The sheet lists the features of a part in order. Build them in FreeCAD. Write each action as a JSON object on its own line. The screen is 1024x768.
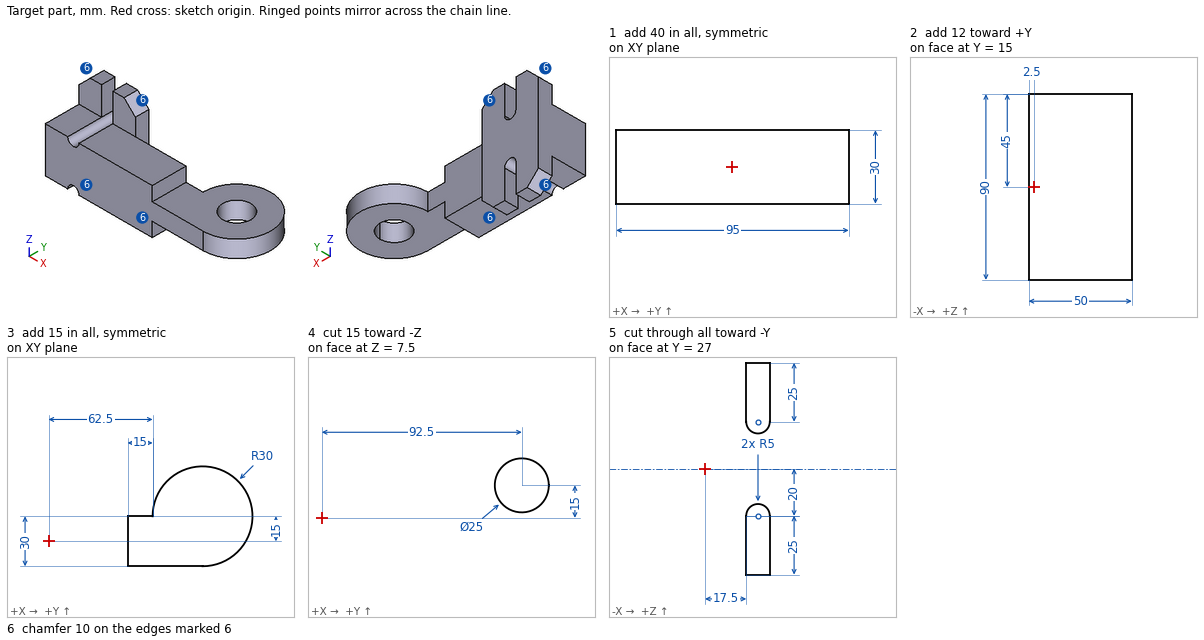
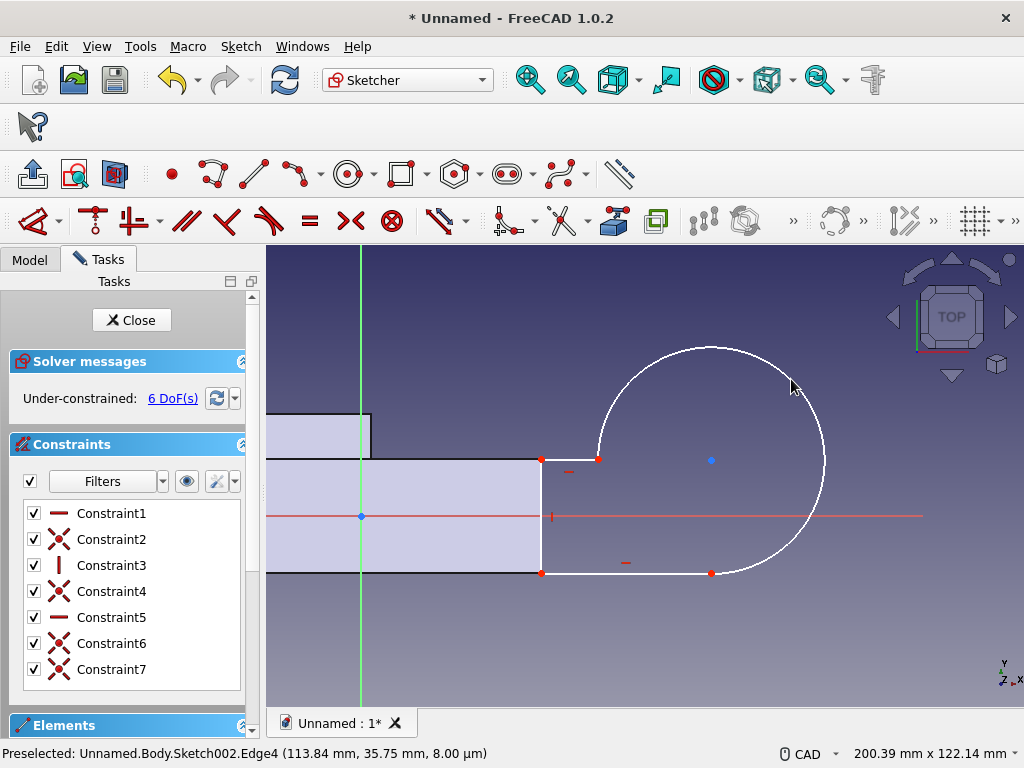
{"action": "left_click", "coordinate": [592, 574]}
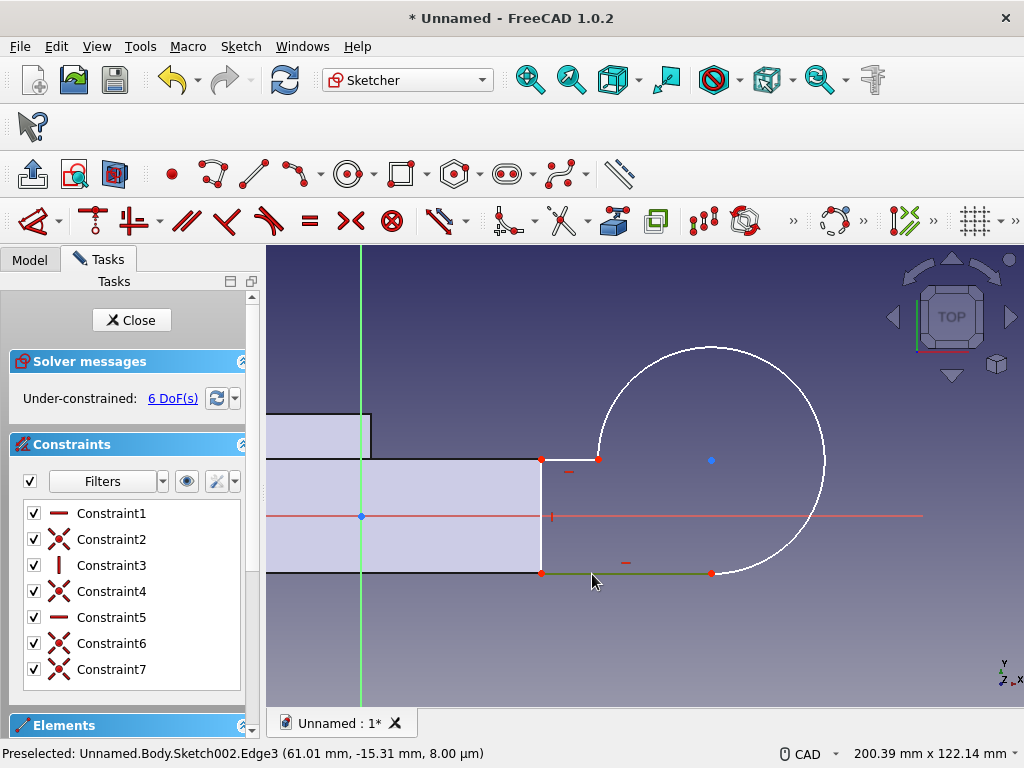
{"action": "left_click", "coordinate": [823, 479]}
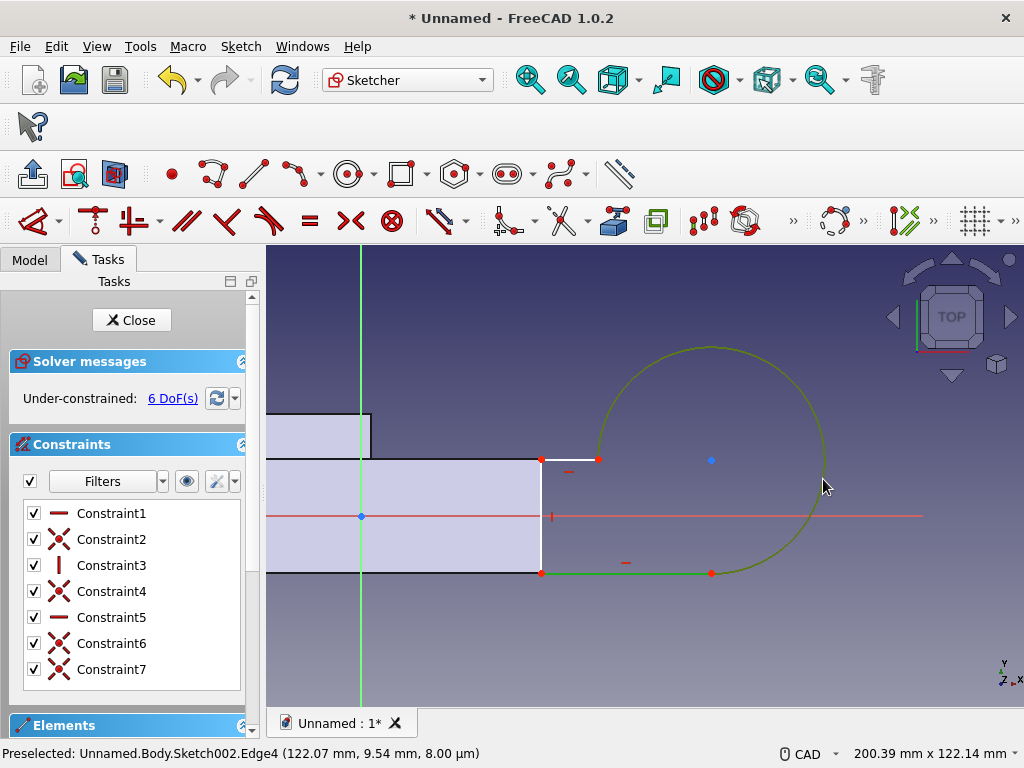
{"action": "left_click", "coordinate": [269, 222]}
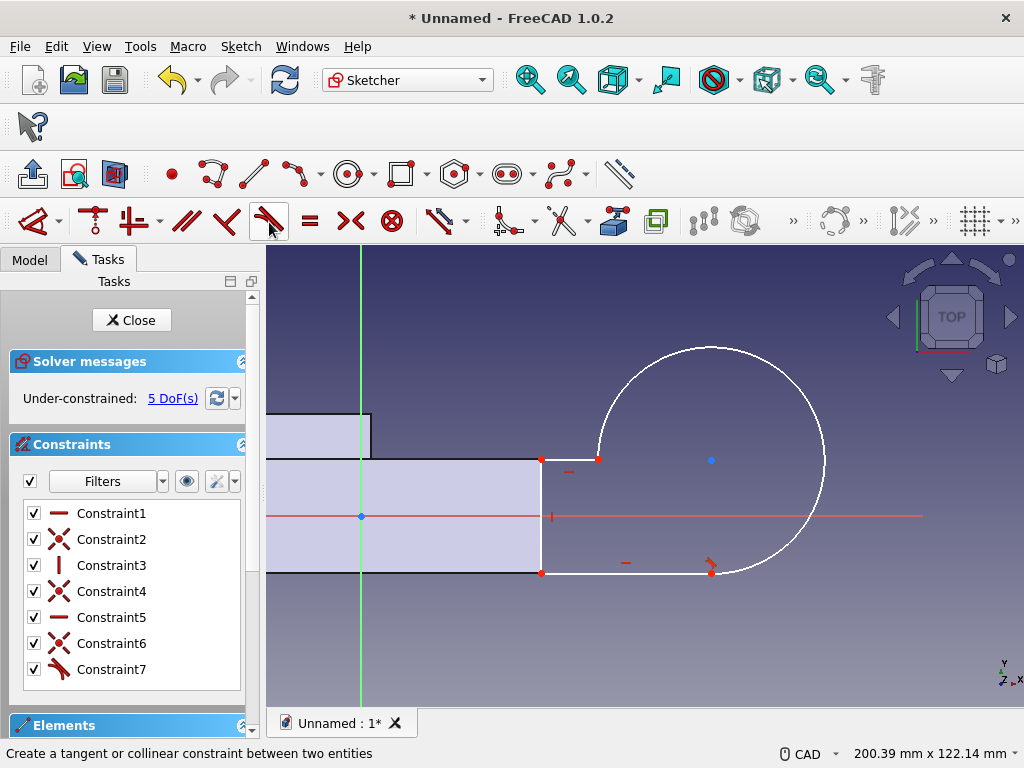
{"action": "left_click", "coordinate": [32, 222]}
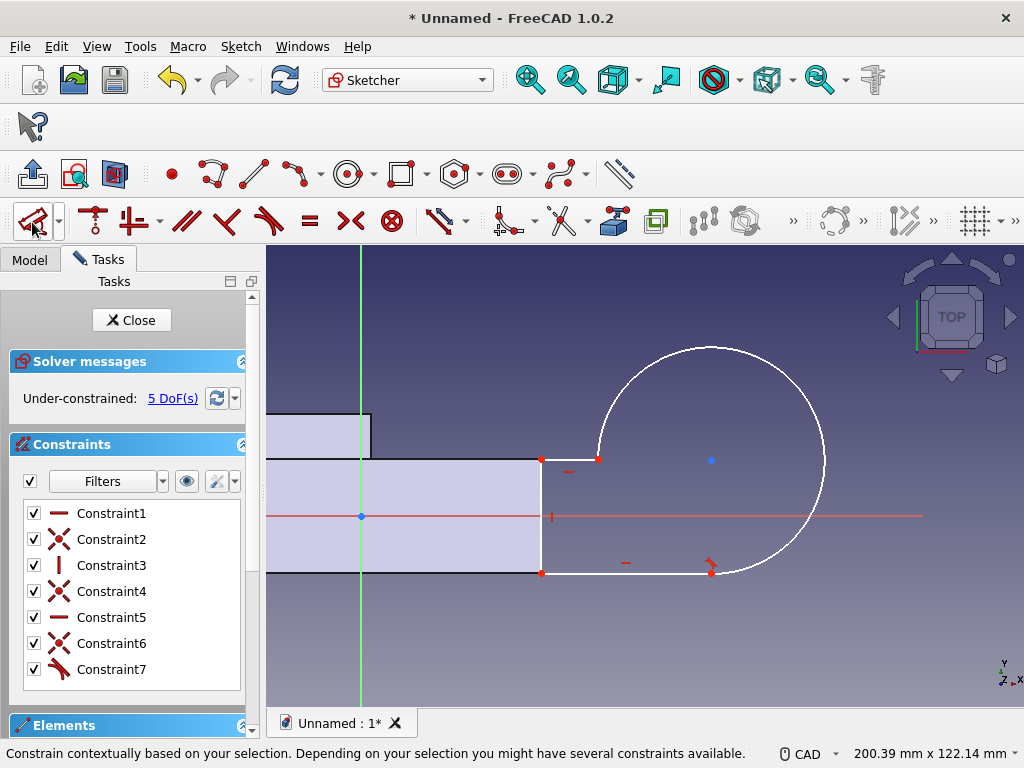
{"action": "left_click", "coordinate": [823, 479]}
{"action": "left_click", "coordinate": [855, 484]}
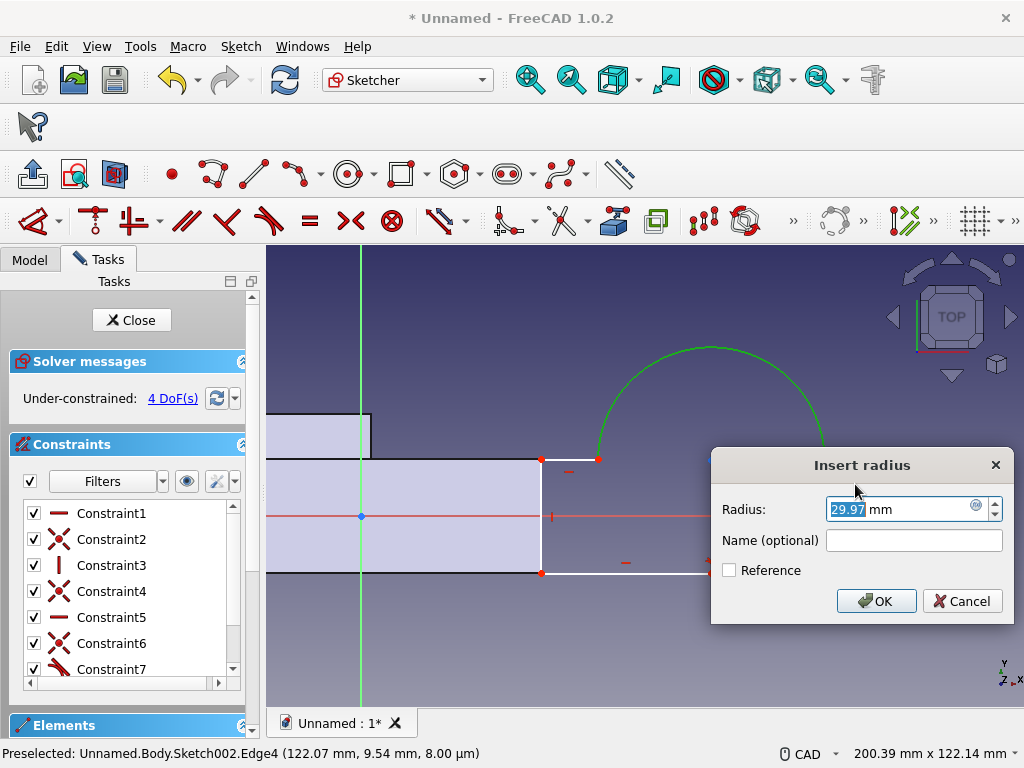
{"action": "type", "text": "30"}
{"action": "key", "text": "Return"}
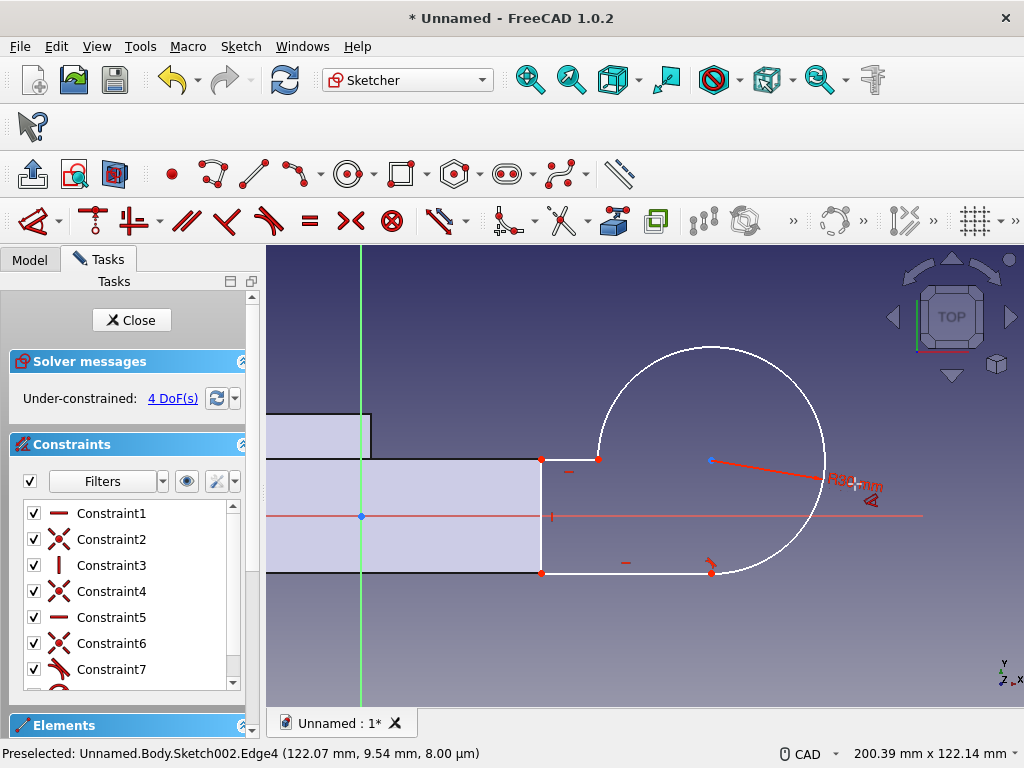
{"action": "left_click", "coordinate": [581, 460]}
{"action": "left_click", "coordinate": [570, 426]}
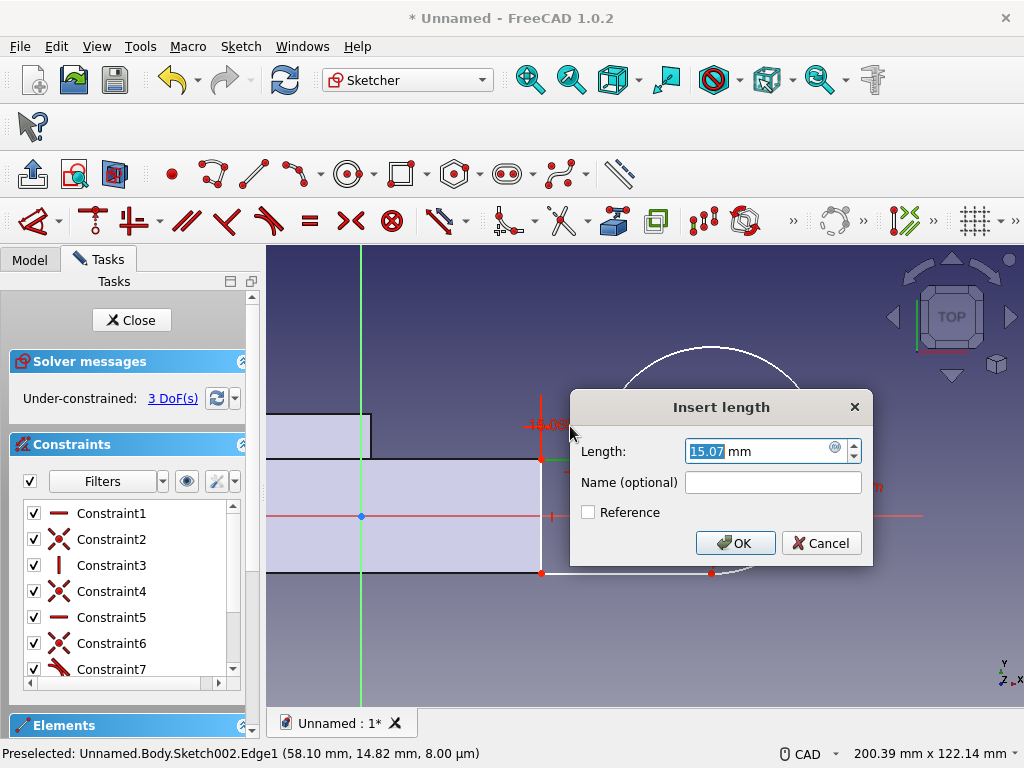
{"action": "type", "text": "15"}
{"action": "key", "text": "Return"}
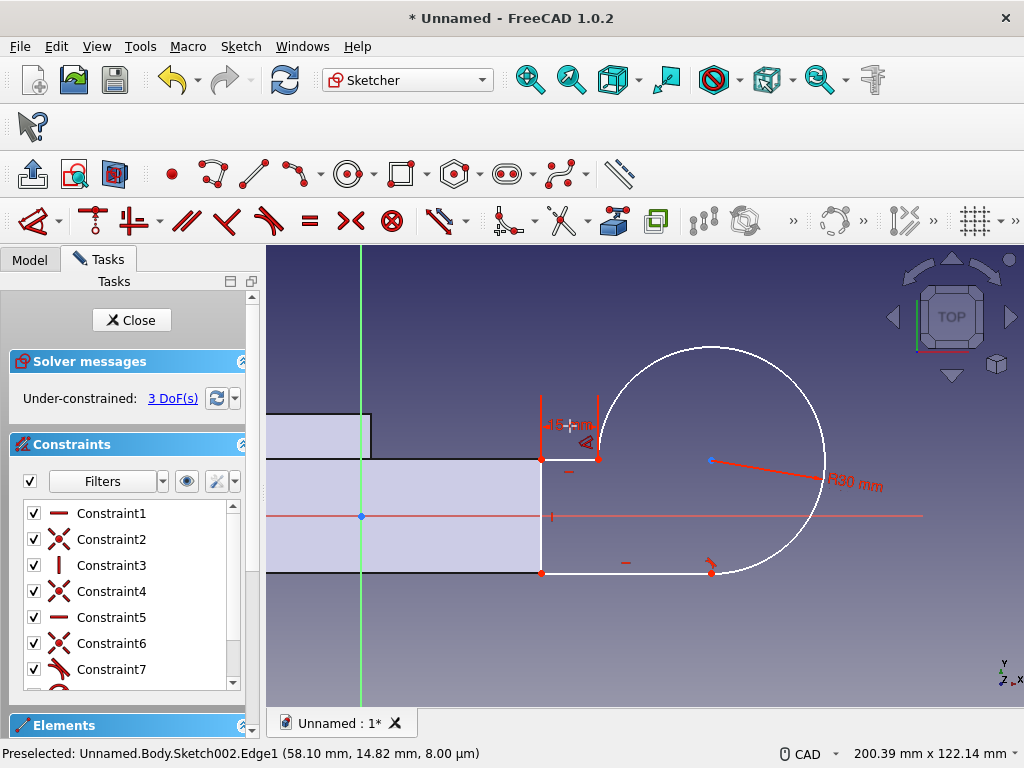
{"action": "left_click", "coordinate": [541, 494]}
{"action": "left_click", "coordinate": [507, 491]}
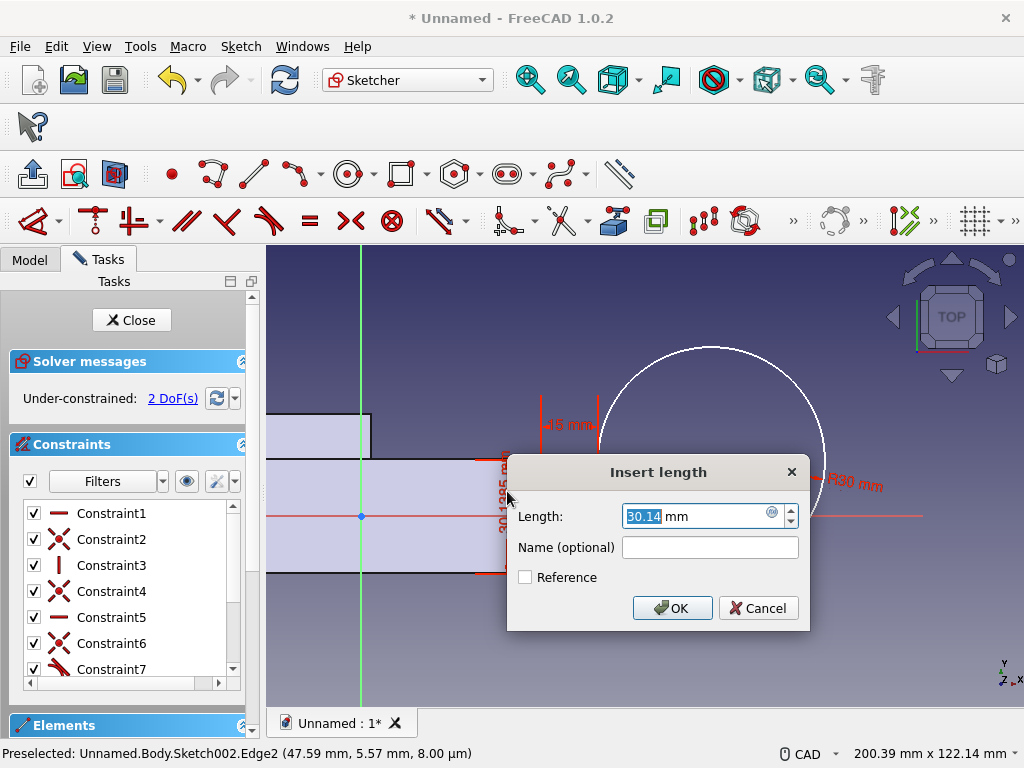
{"action": "type", "text": "30"}
{"action": "key", "text": "Return"}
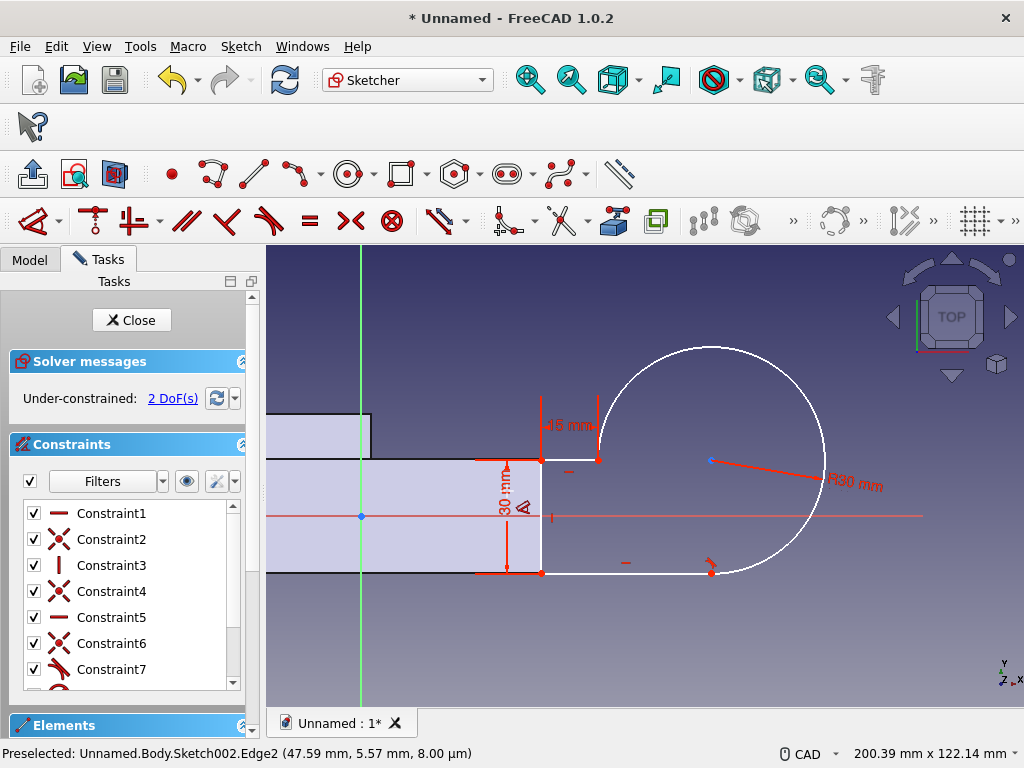
{"action": "left_click", "coordinate": [598, 460]}
{"action": "left_click", "coordinate": [327, 488]}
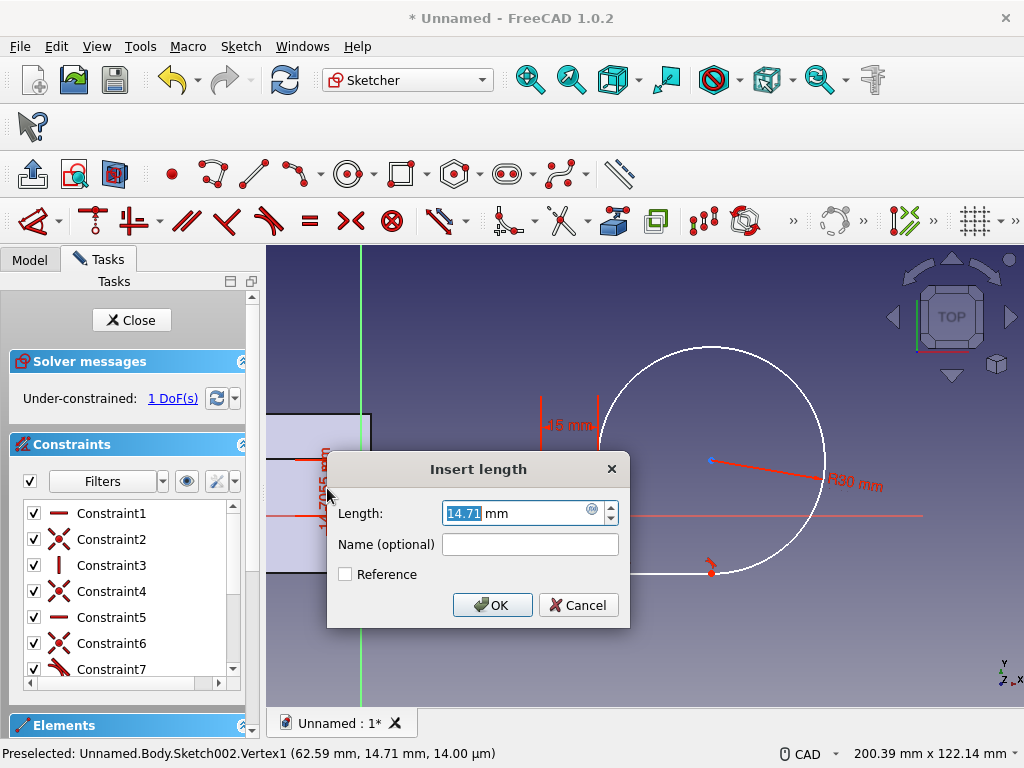
{"action": "type", "text": "15"}
{"action": "key", "text": "Return"}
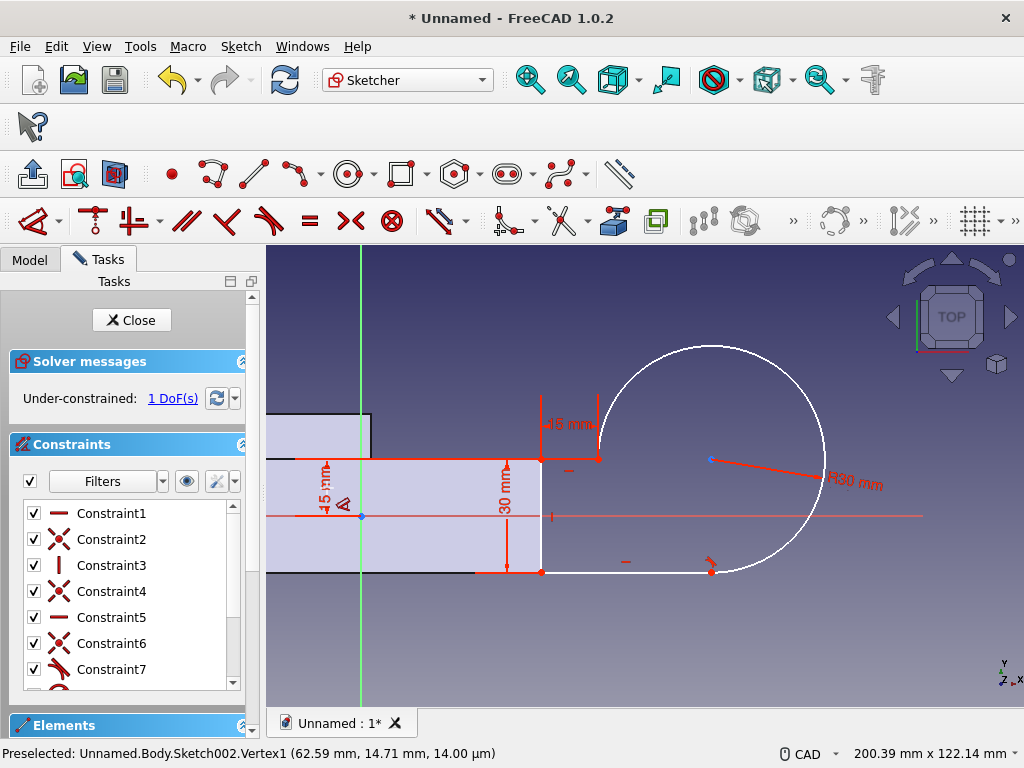
{"action": "left_click", "coordinate": [598, 459]}
{"action": "left_click", "coordinate": [480, 550]}